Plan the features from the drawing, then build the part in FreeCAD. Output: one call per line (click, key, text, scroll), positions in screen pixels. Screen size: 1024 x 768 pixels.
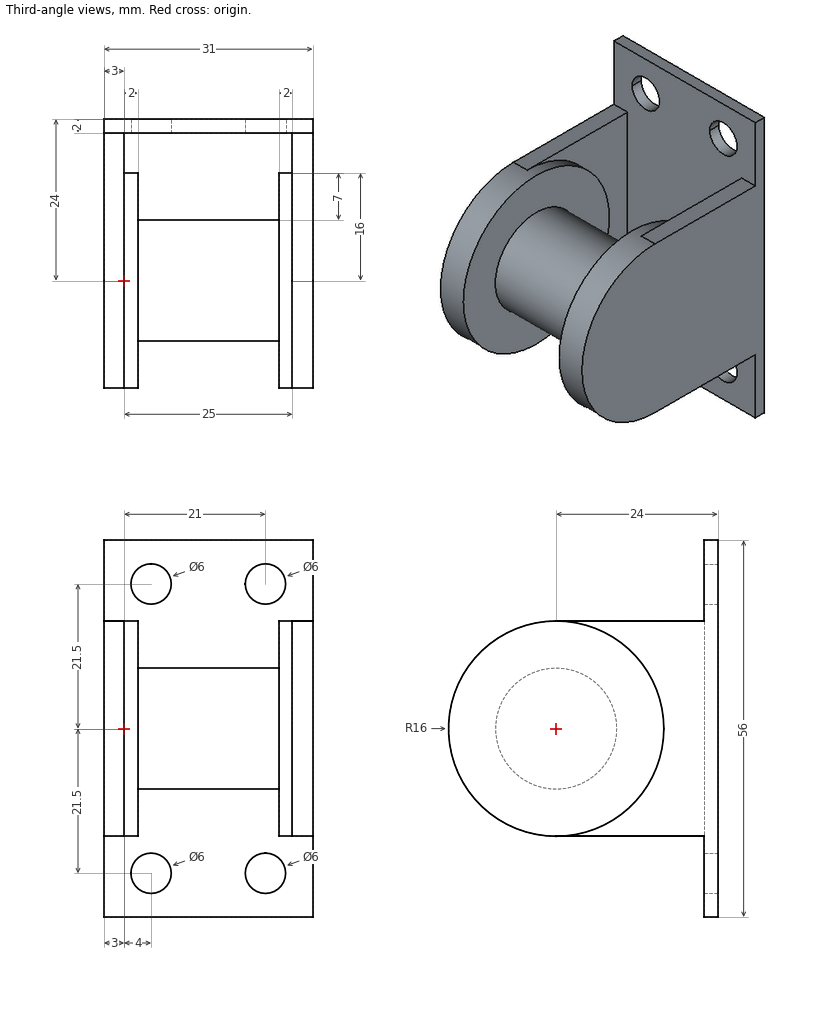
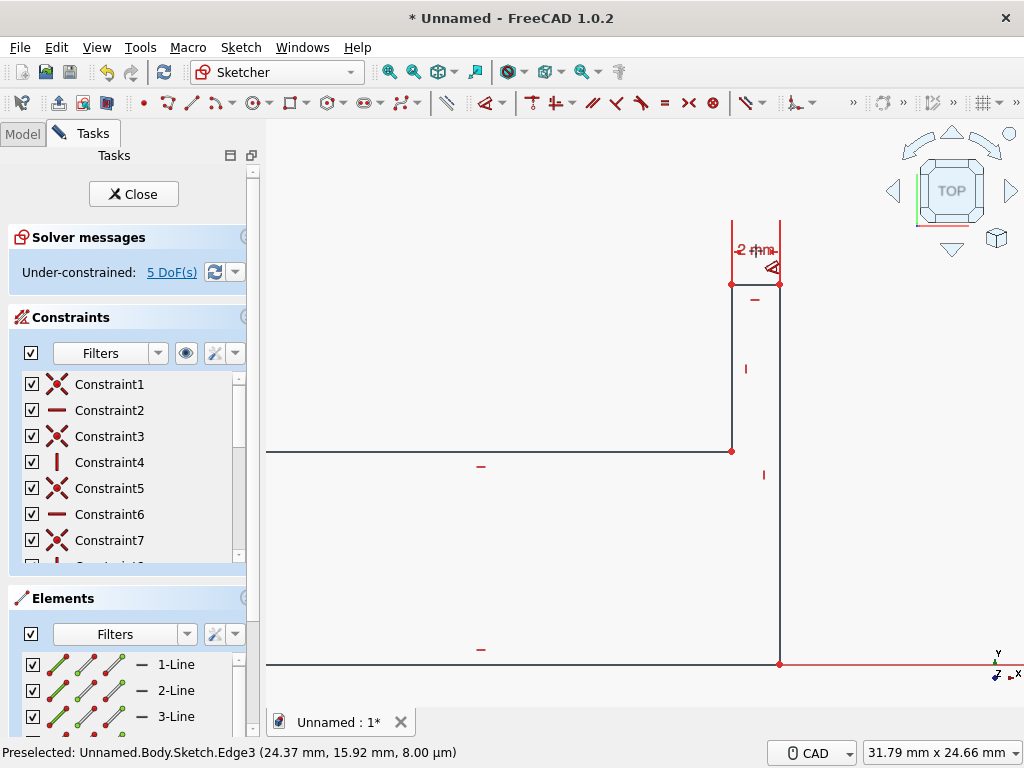
click(732, 335)
click(766, 368)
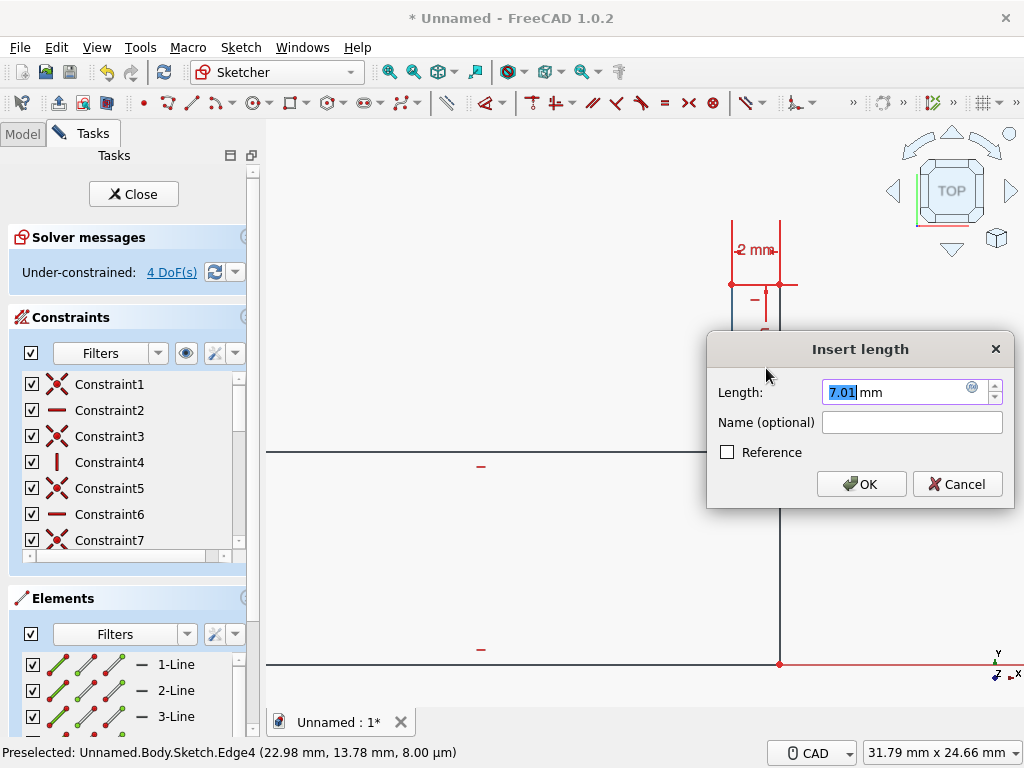
text(7)
key(Return)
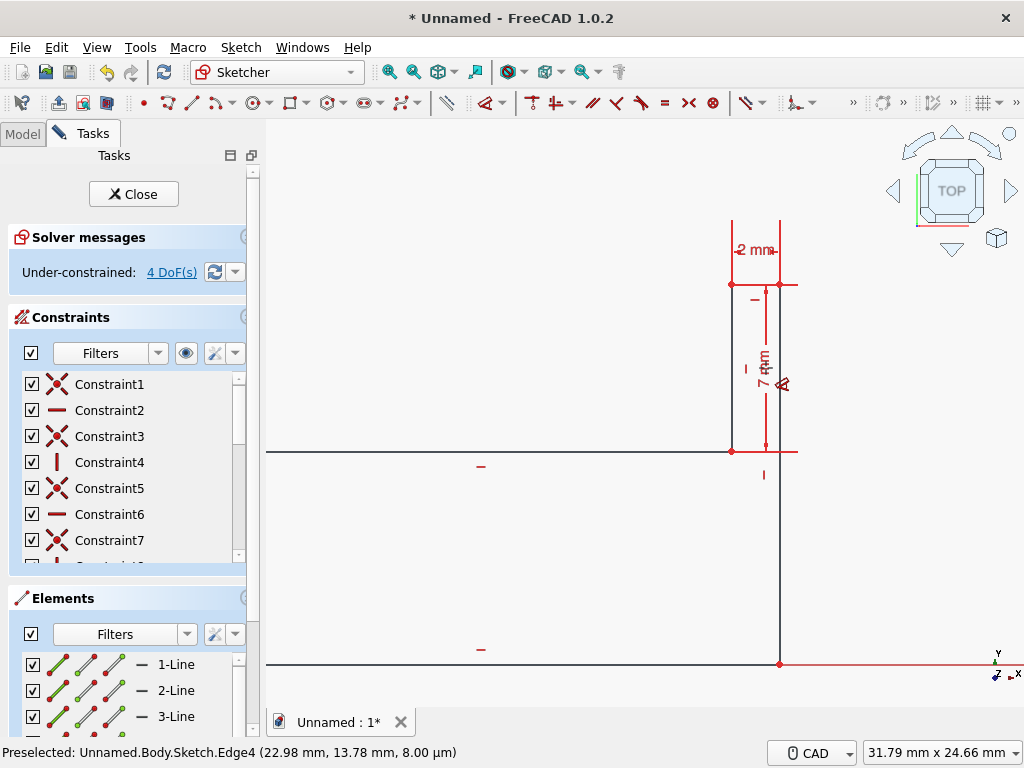
scroll(769, 289, down, 2)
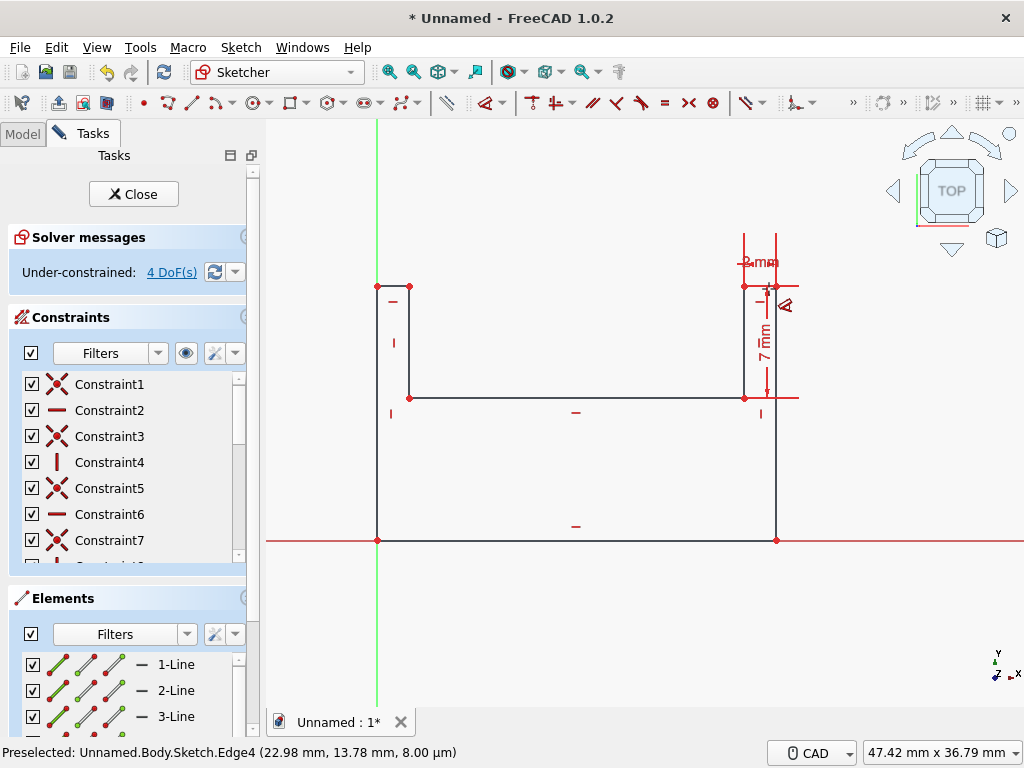
click(409, 365)
click(443, 342)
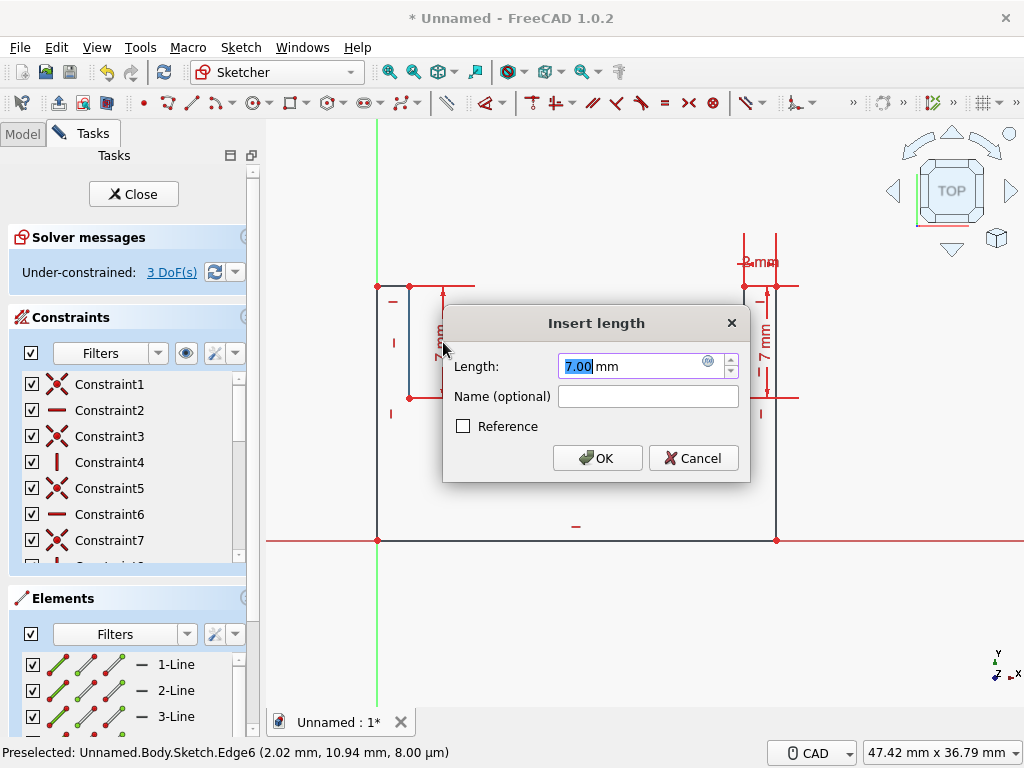
text(7)
key(Return)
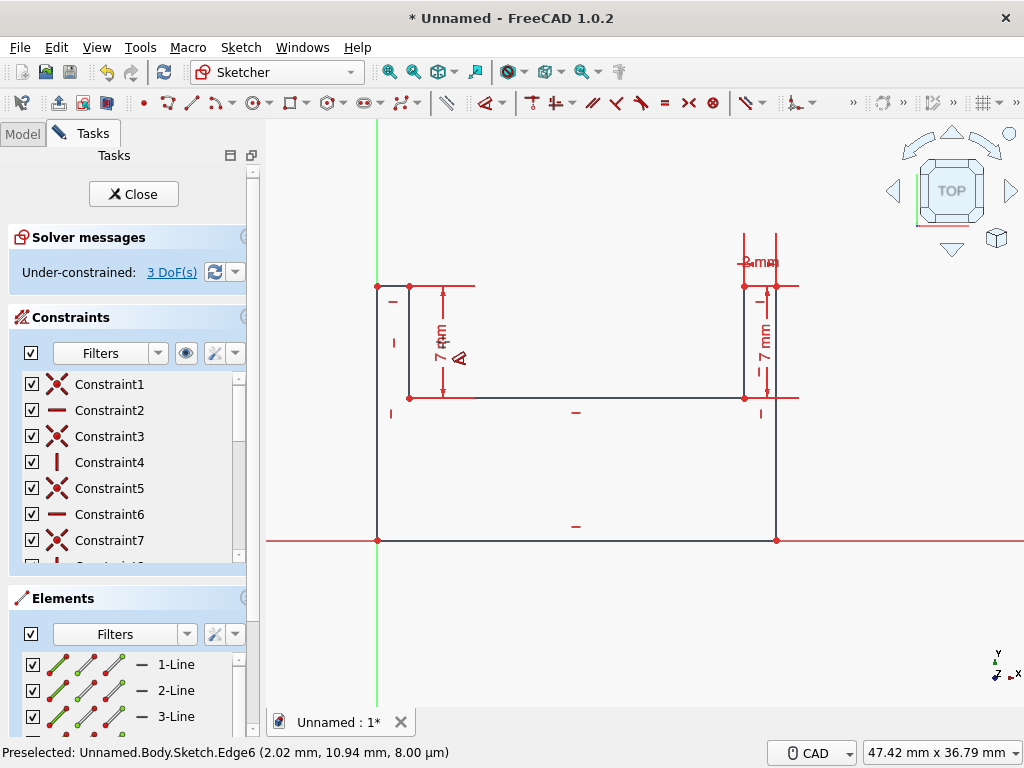
scroll(400, 286, up, 2)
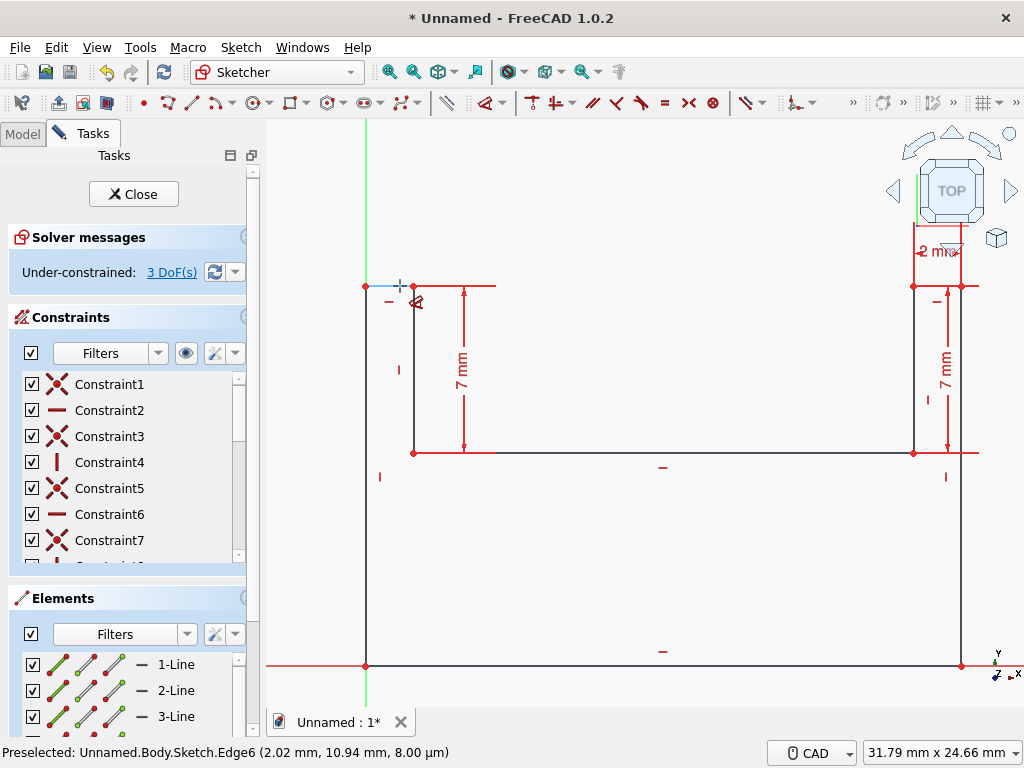
click(399, 286)
click(390, 252)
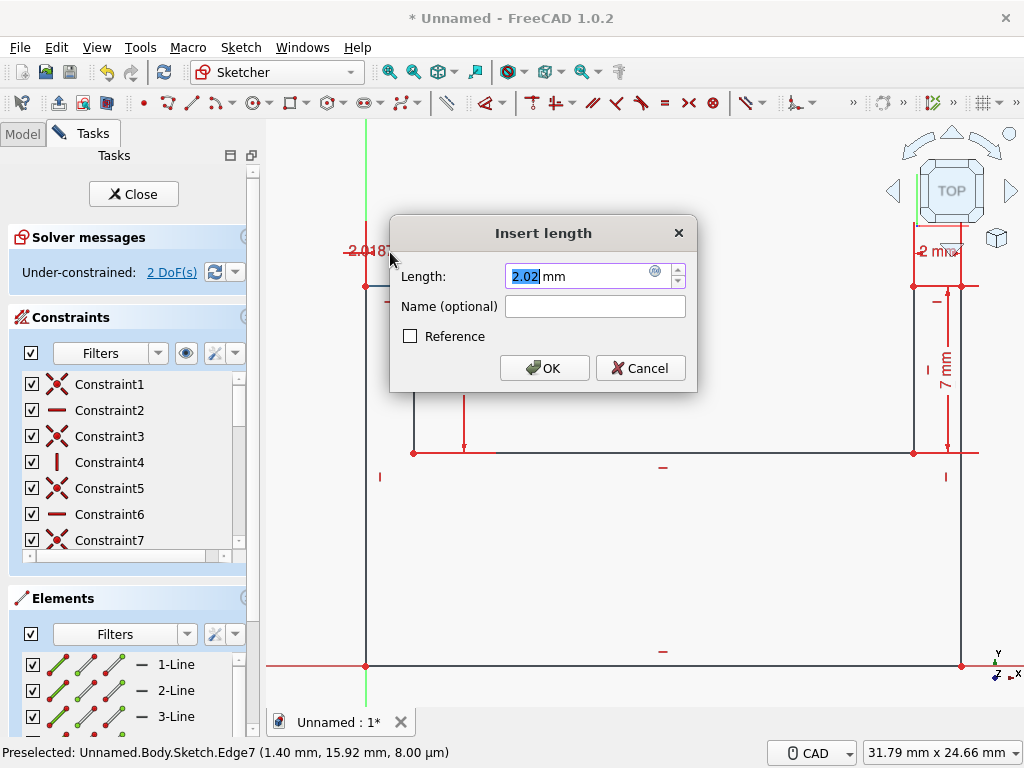
text(2)
key(Return)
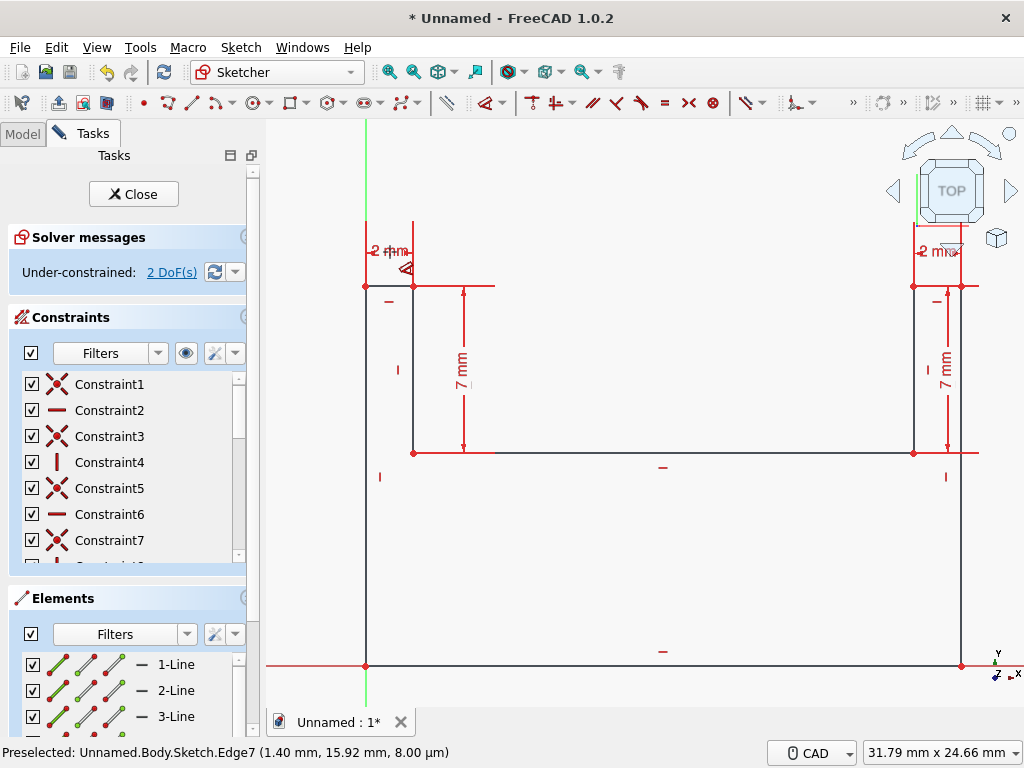
click(544, 666)
click(612, 632)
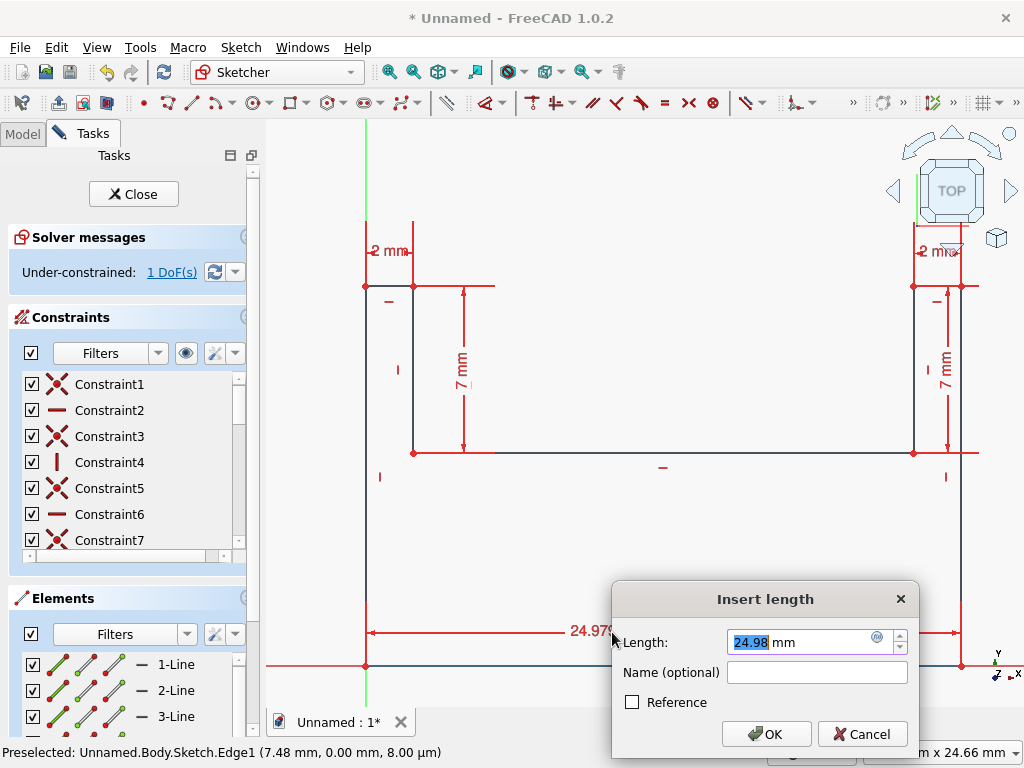
text(25)
key(Return)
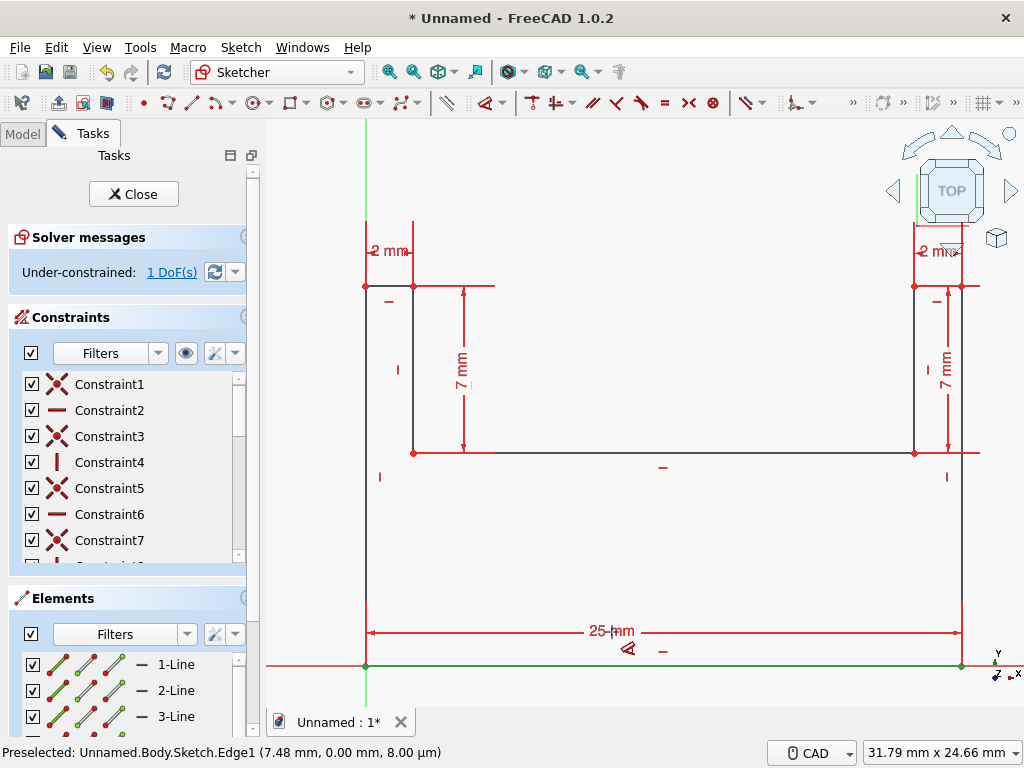
scroll(399, 286, down, 2)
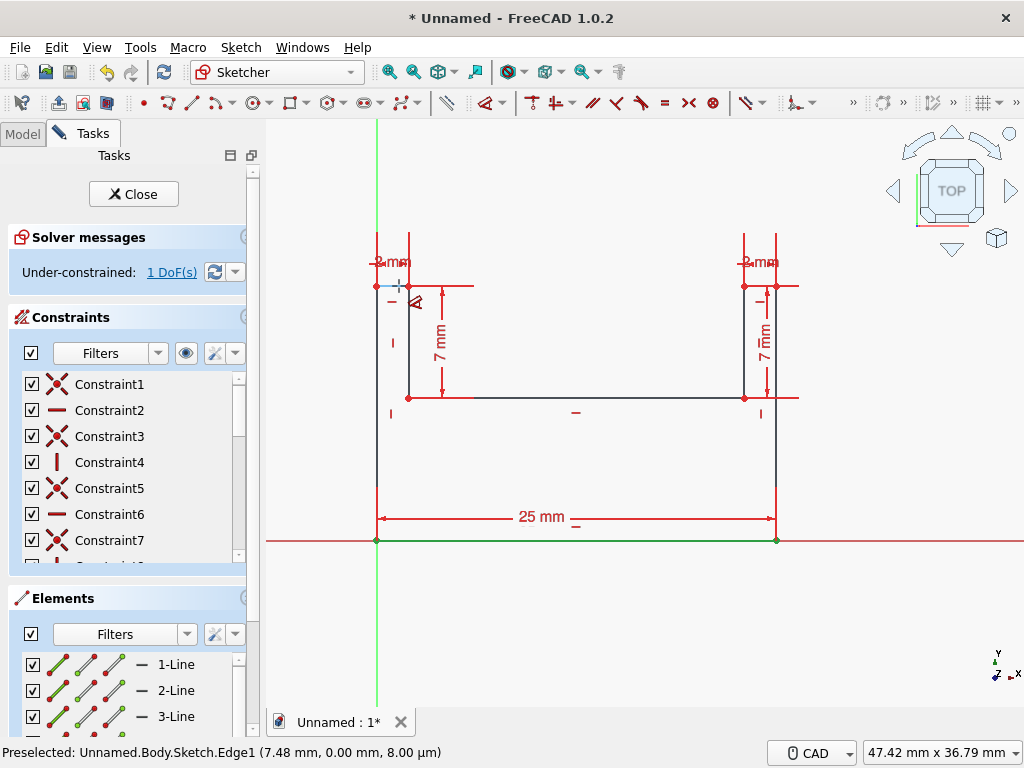
click(776, 464)
click(810, 414)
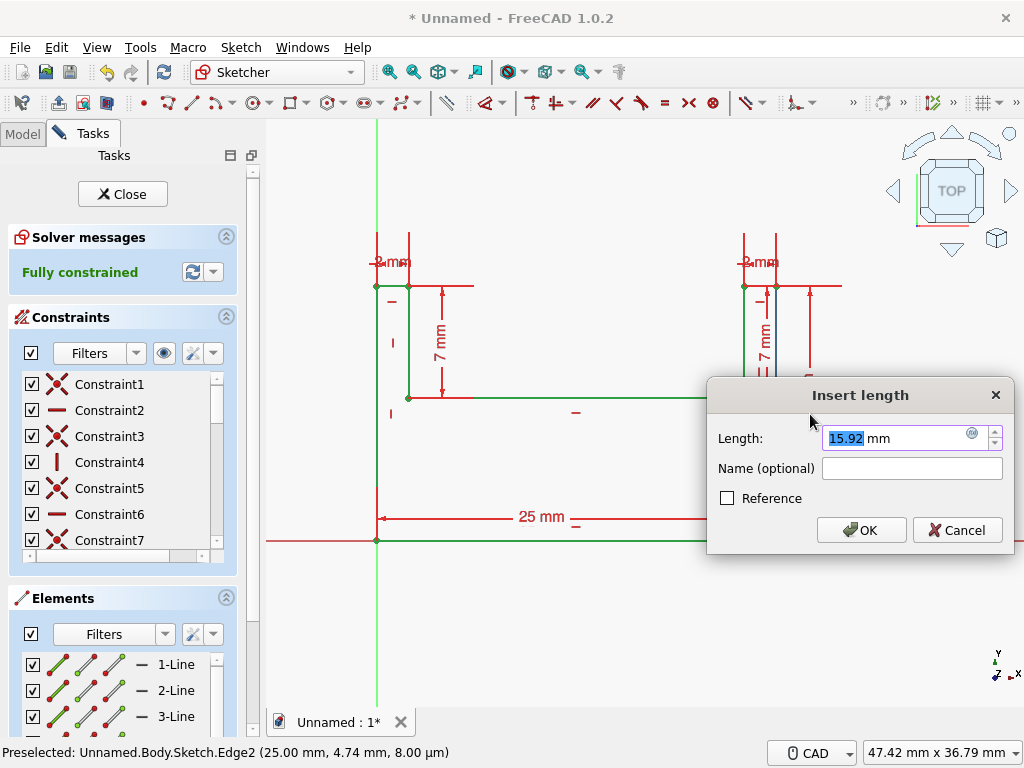
text(16)
key(Return)
key(Escape)